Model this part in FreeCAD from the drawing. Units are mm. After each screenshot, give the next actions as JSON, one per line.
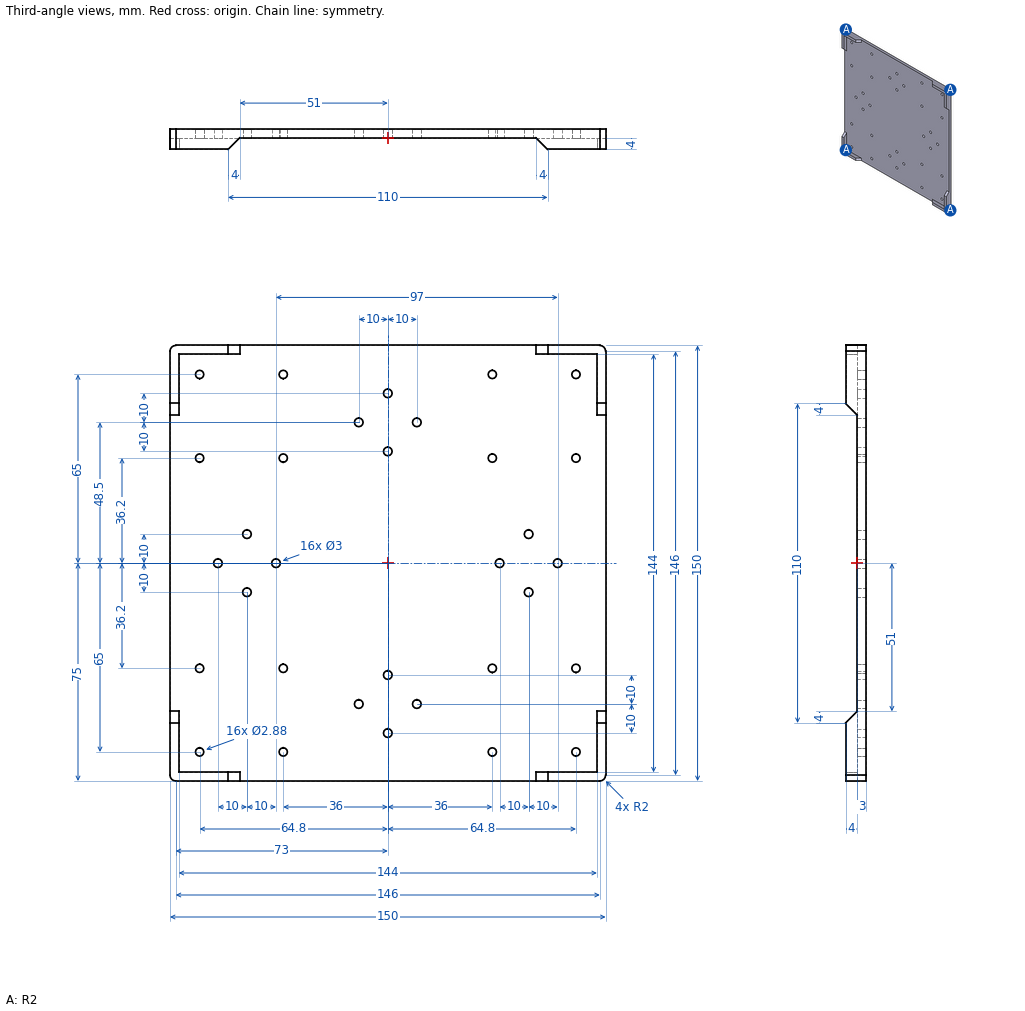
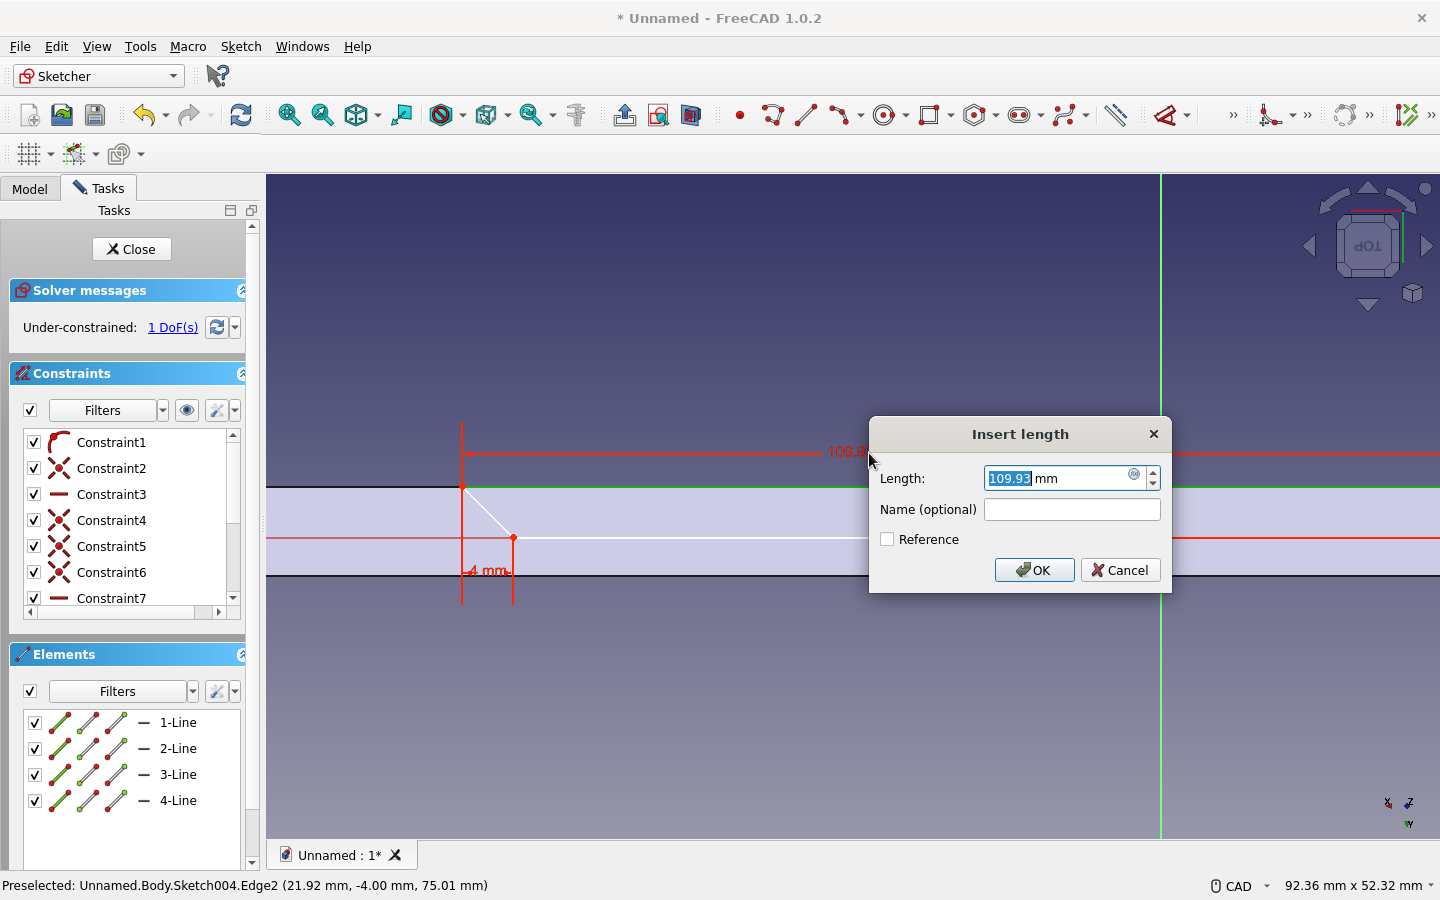
{"action": "type", "text": "110"}
{"action": "key", "text": "Return"}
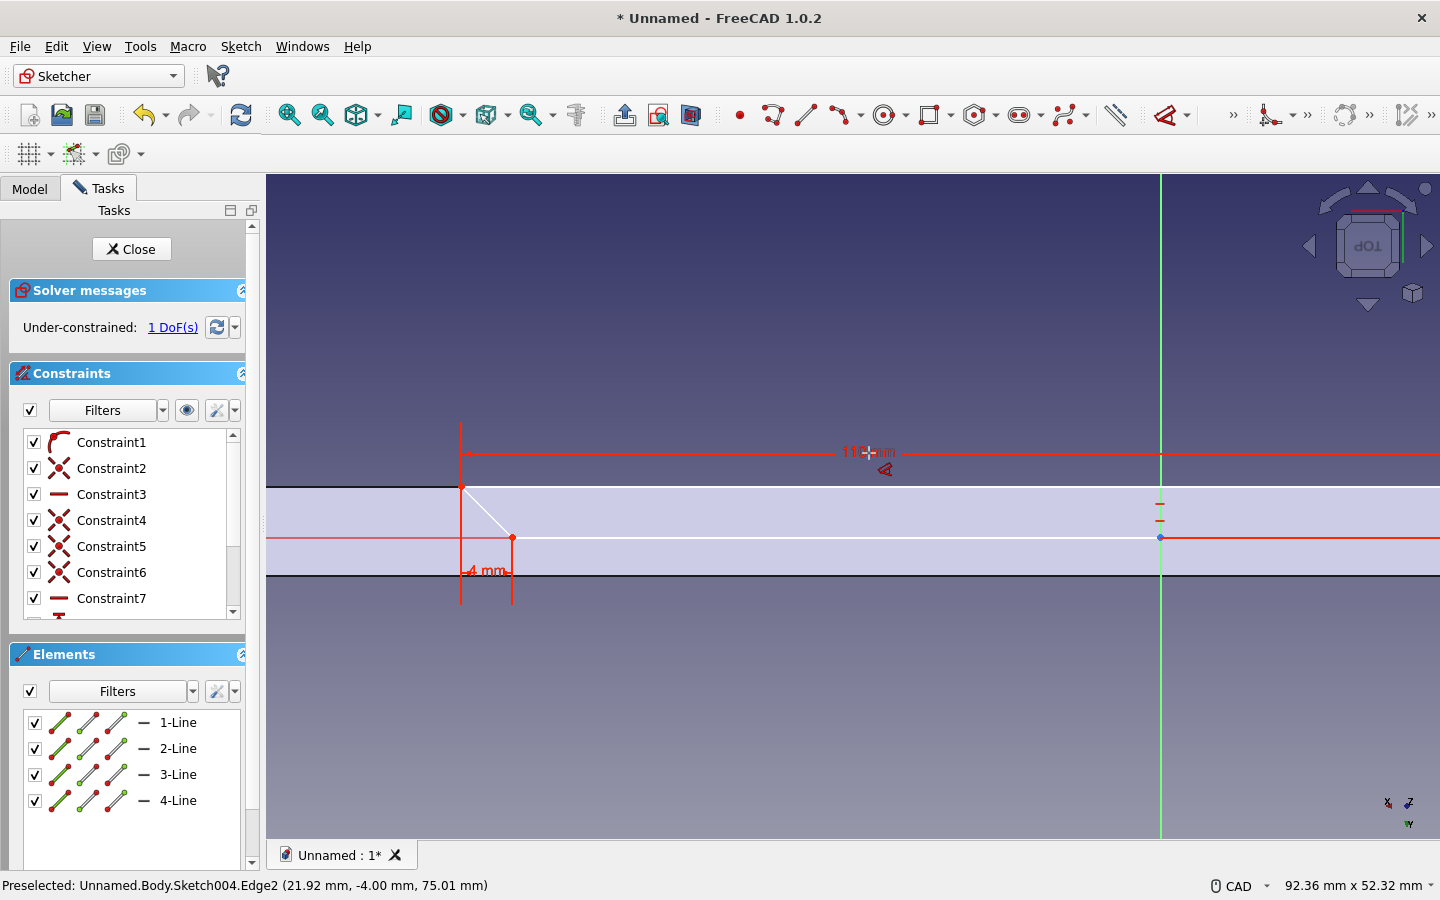
{"action": "scroll", "coordinate": [478, 502], "scroll_direction": "down", "scroll_amount": 4}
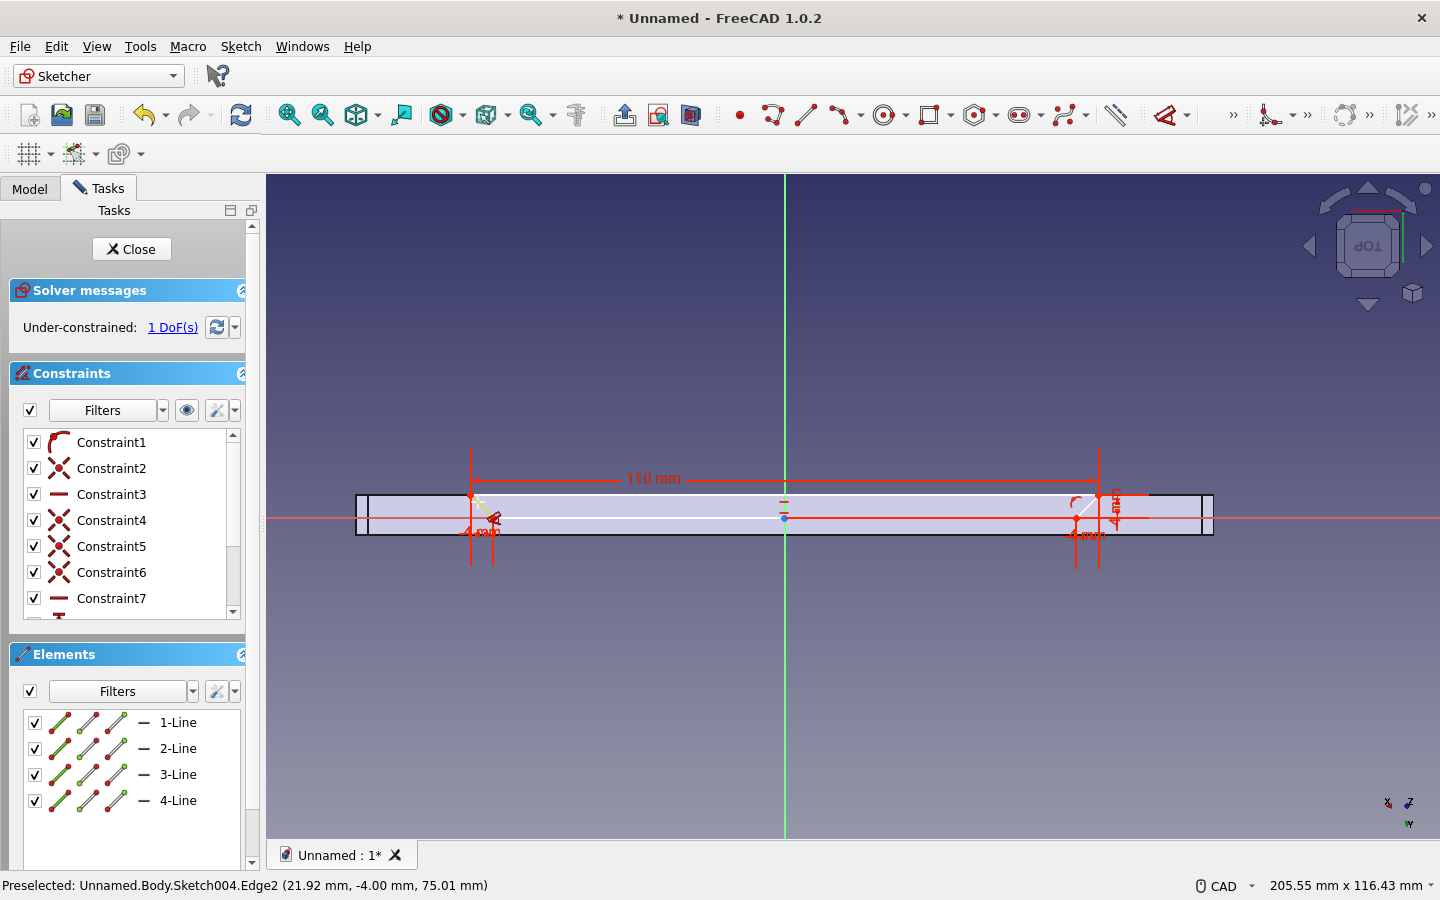
{"action": "left_click", "coordinate": [1076, 518]}
{"action": "left_click", "coordinate": [930, 552]}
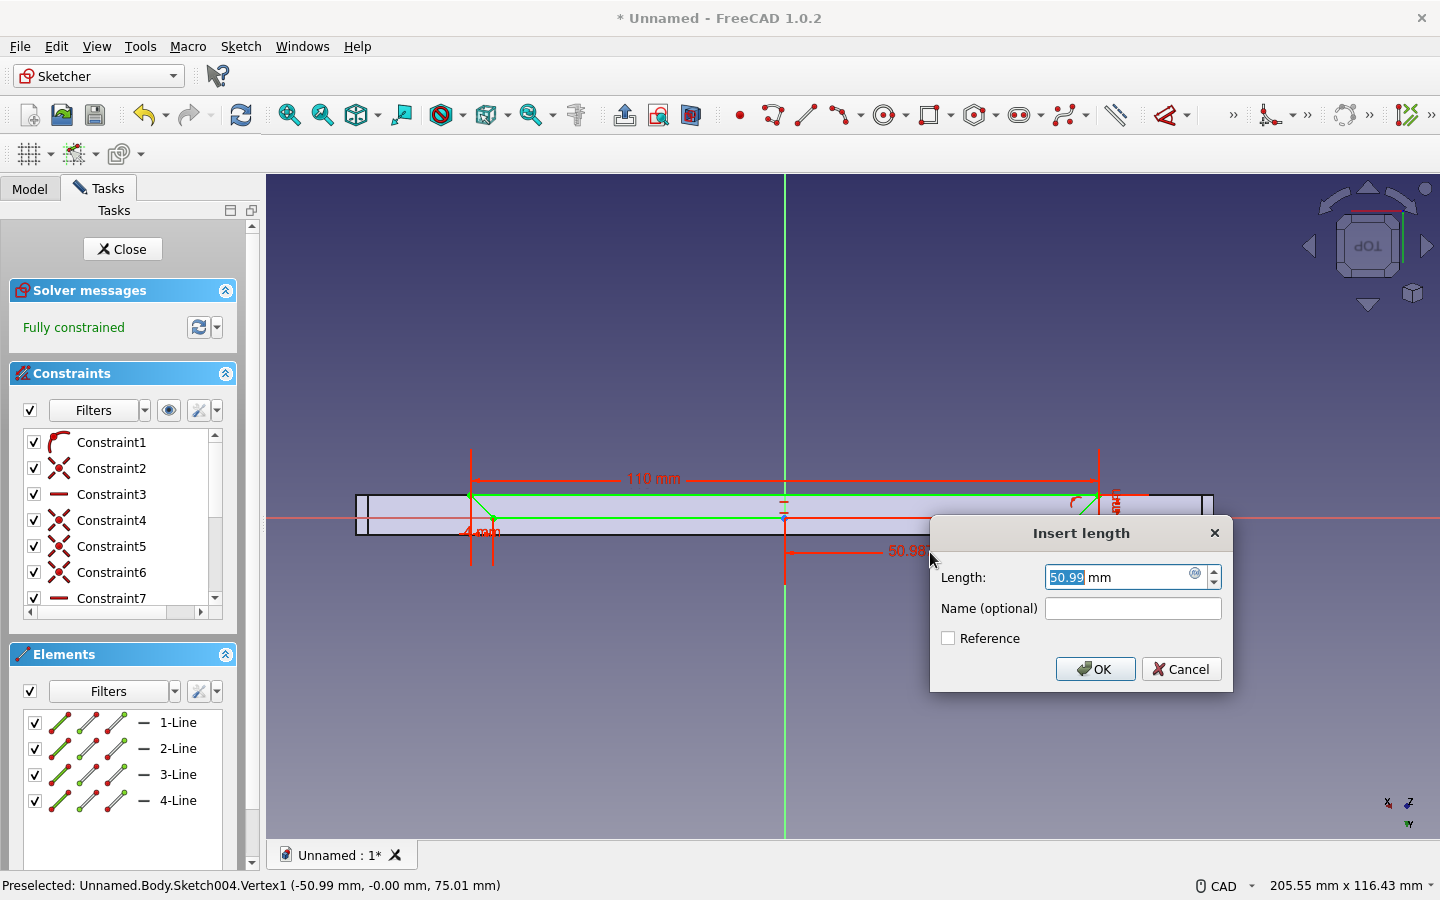
{"action": "type", "text": "51"}
{"action": "key", "text": "Return"}
{"action": "key", "text": "Escape"}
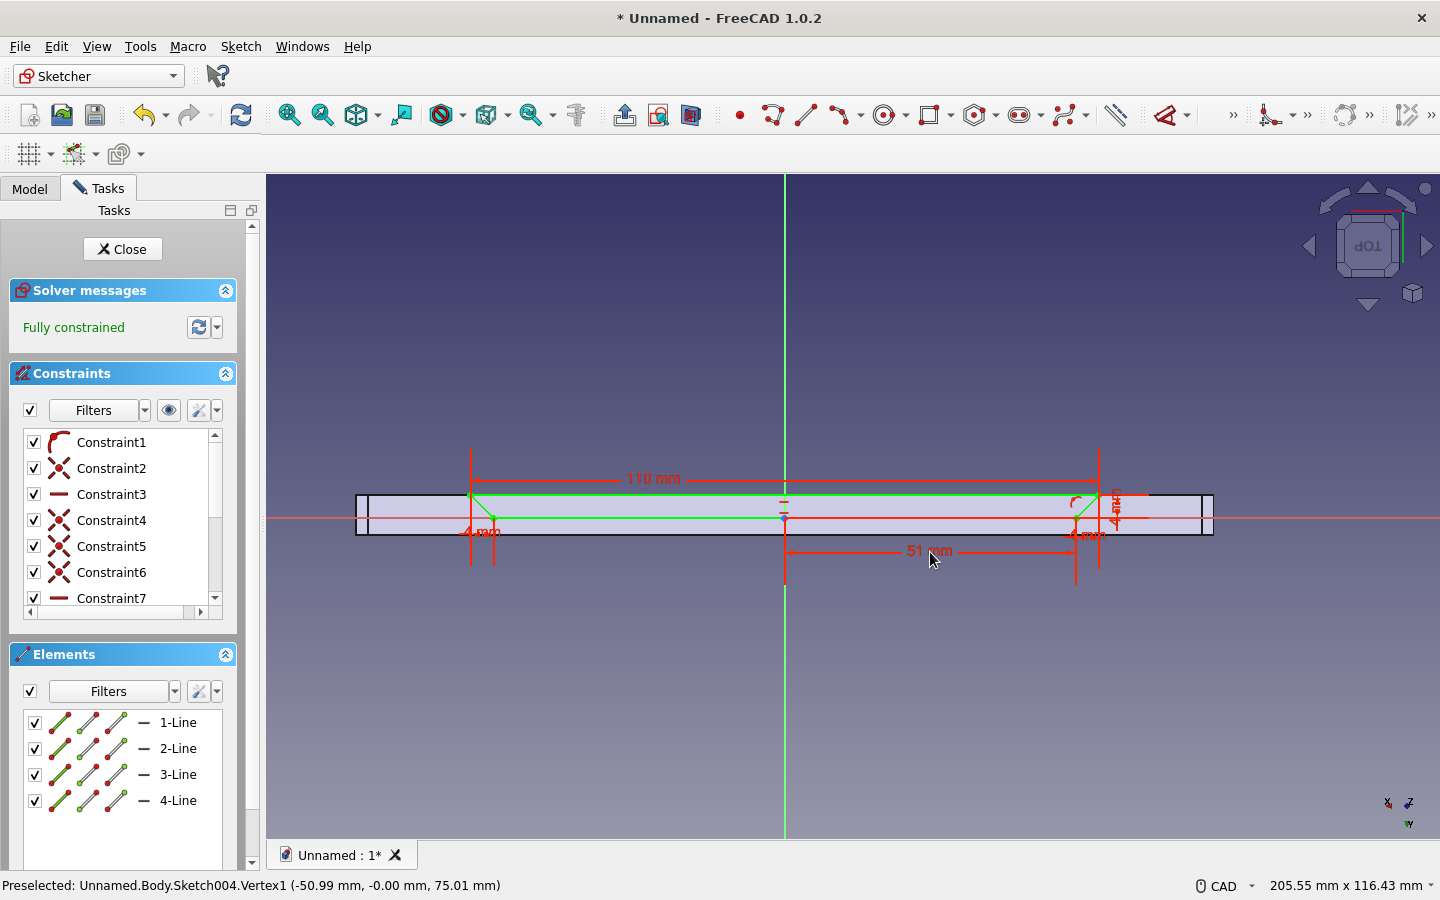
{"action": "left_click", "coordinate": [123, 249]}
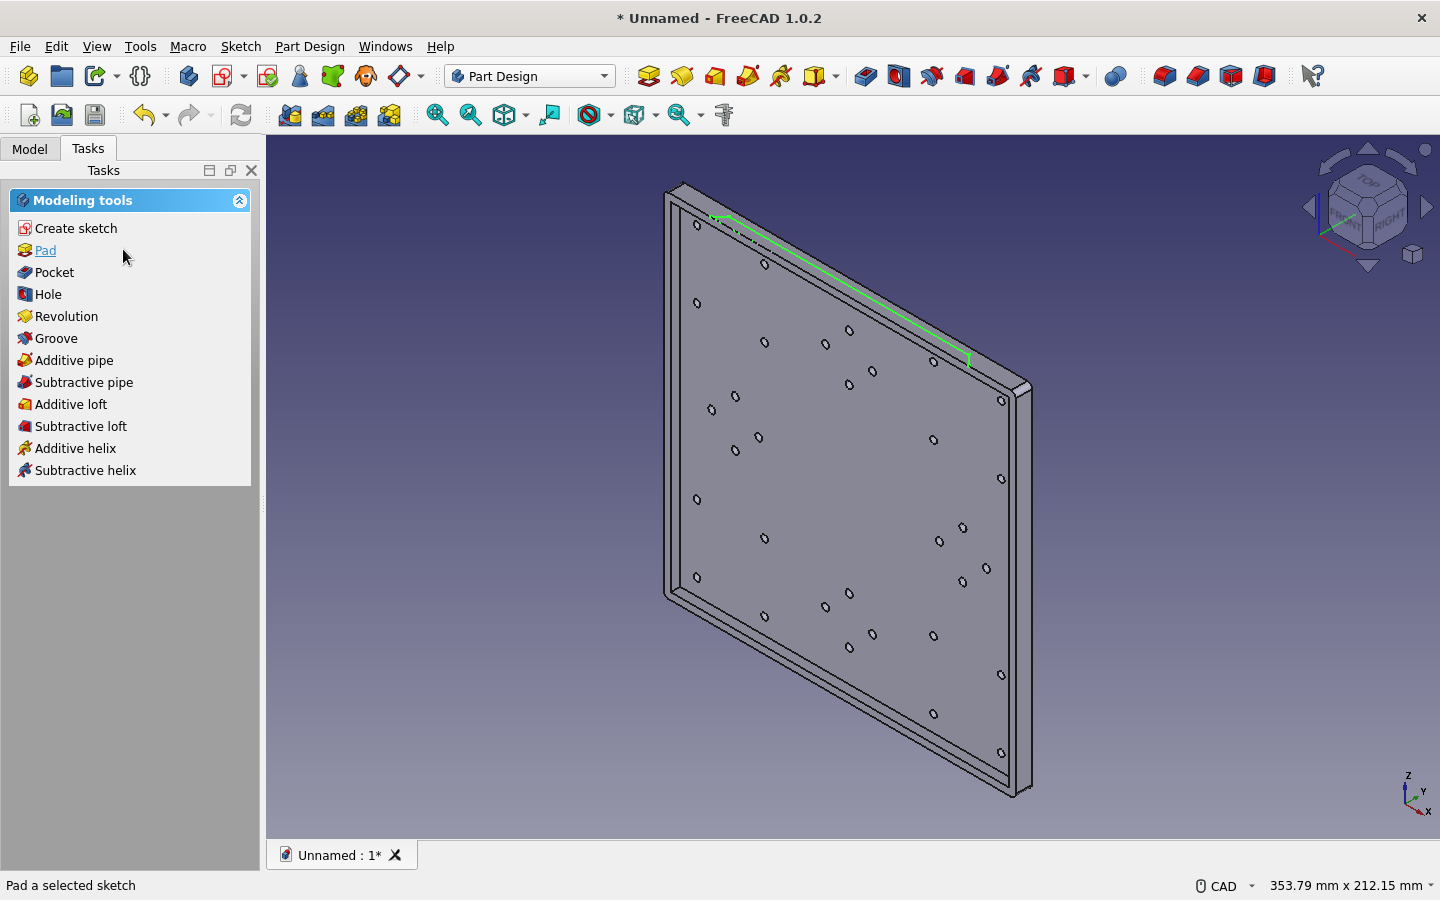
{"action": "left_click", "coordinate": [866, 76]}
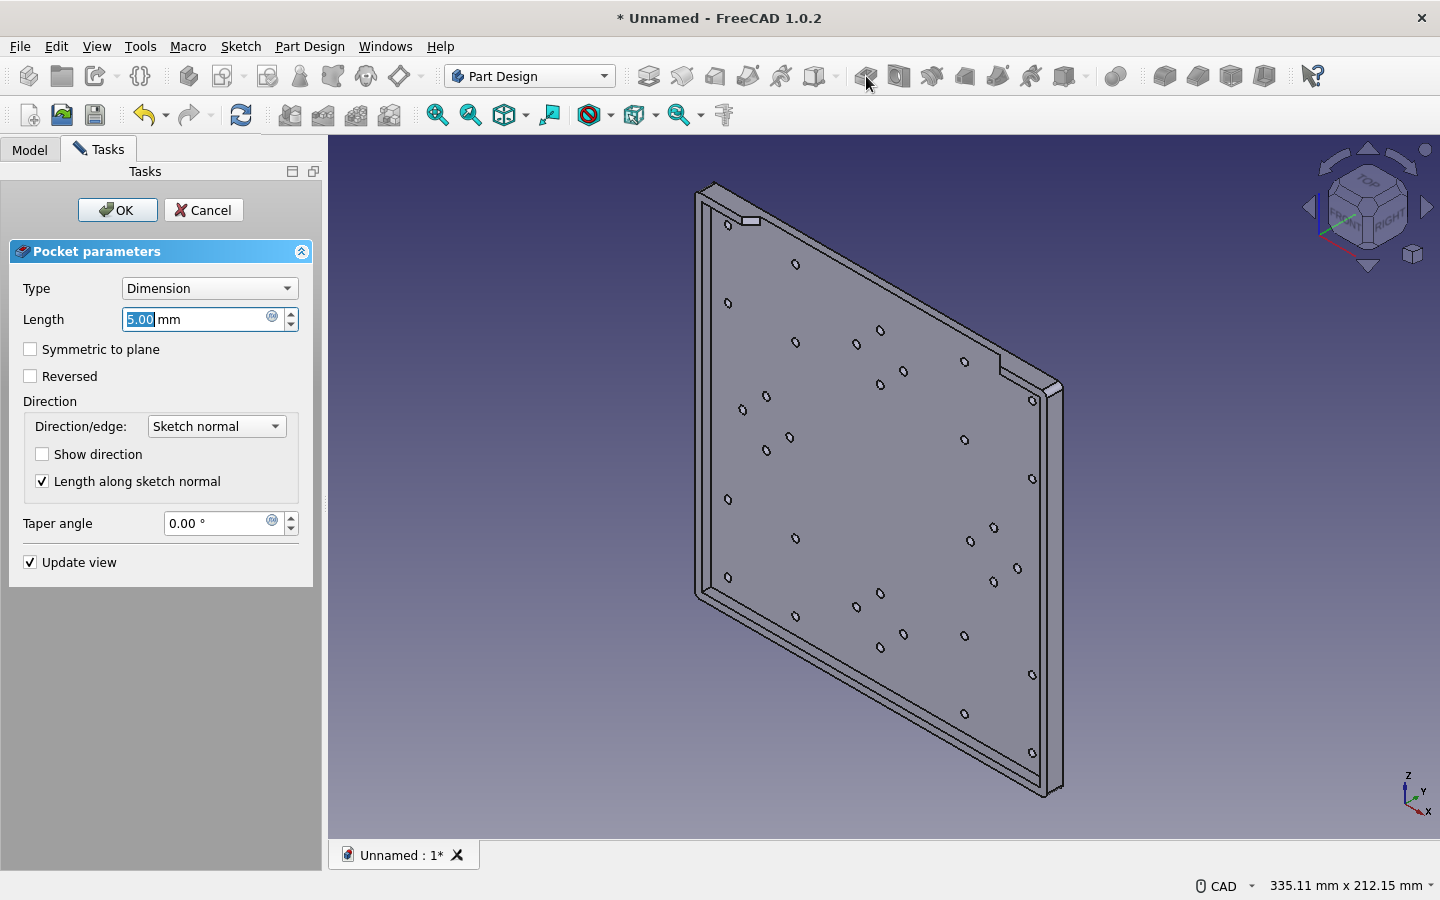
{"action": "left_click", "coordinate": [210, 288]}